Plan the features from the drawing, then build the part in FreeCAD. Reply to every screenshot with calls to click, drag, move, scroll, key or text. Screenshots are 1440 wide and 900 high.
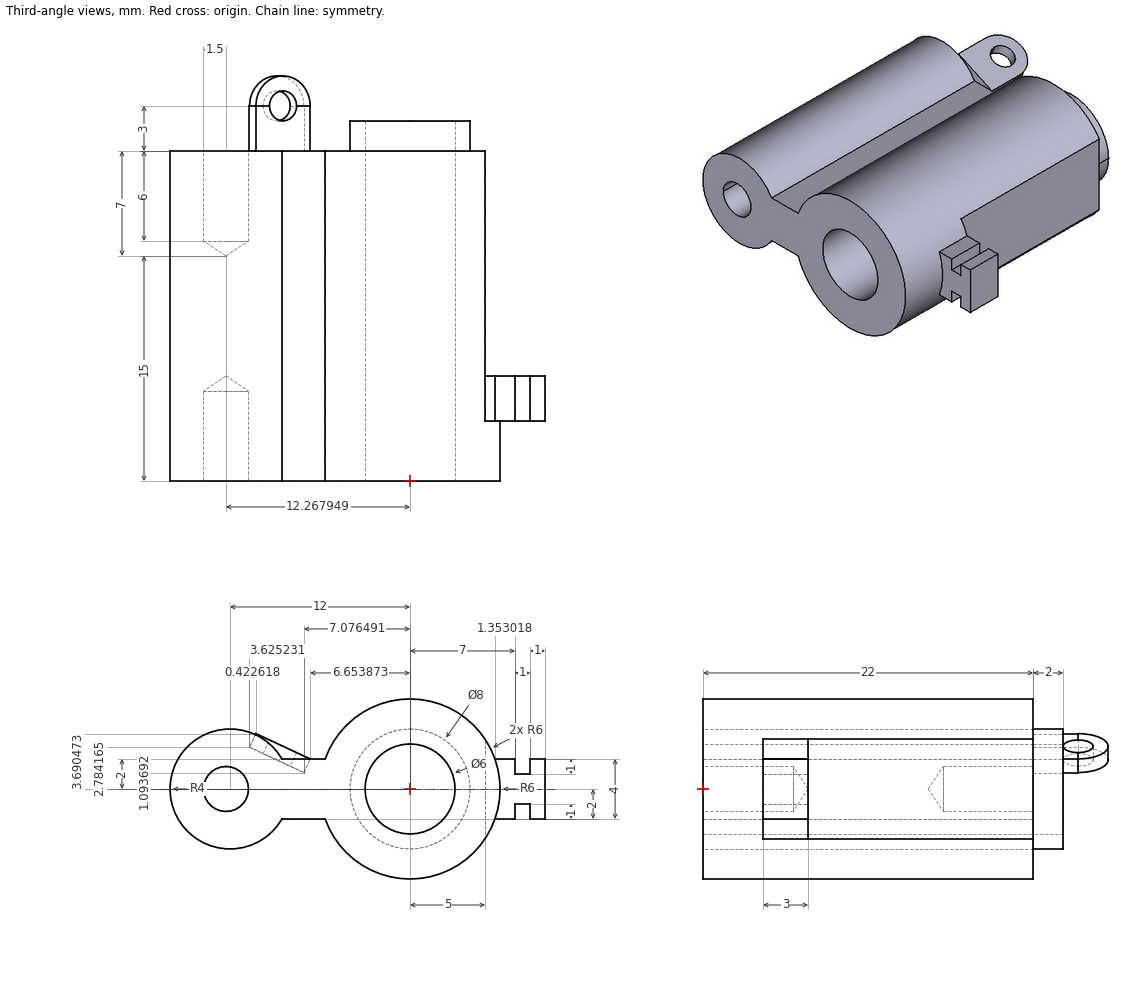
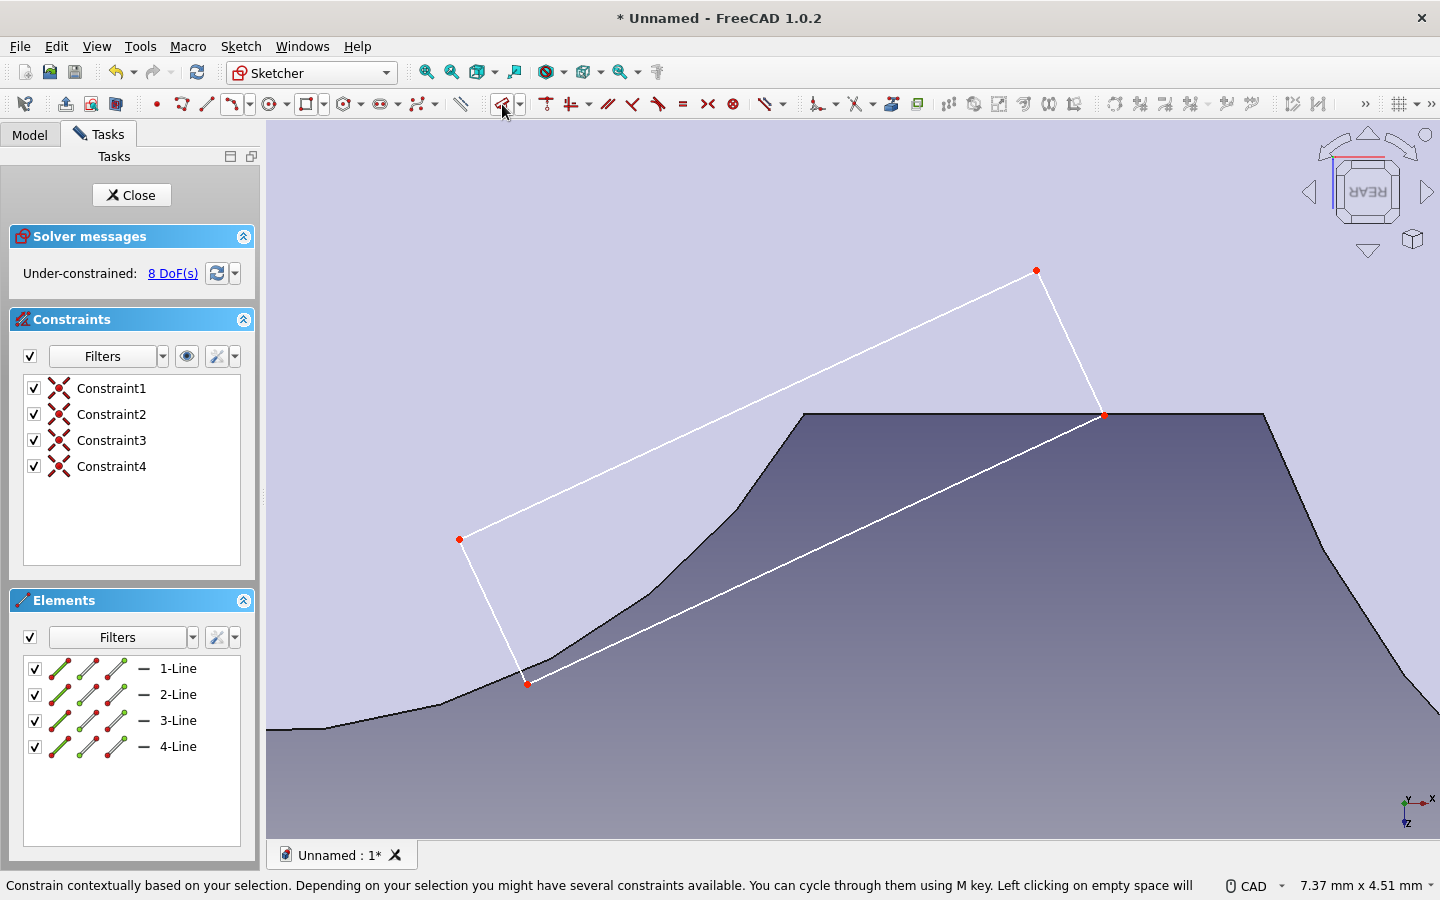
click(1104, 415)
click(1070, 282)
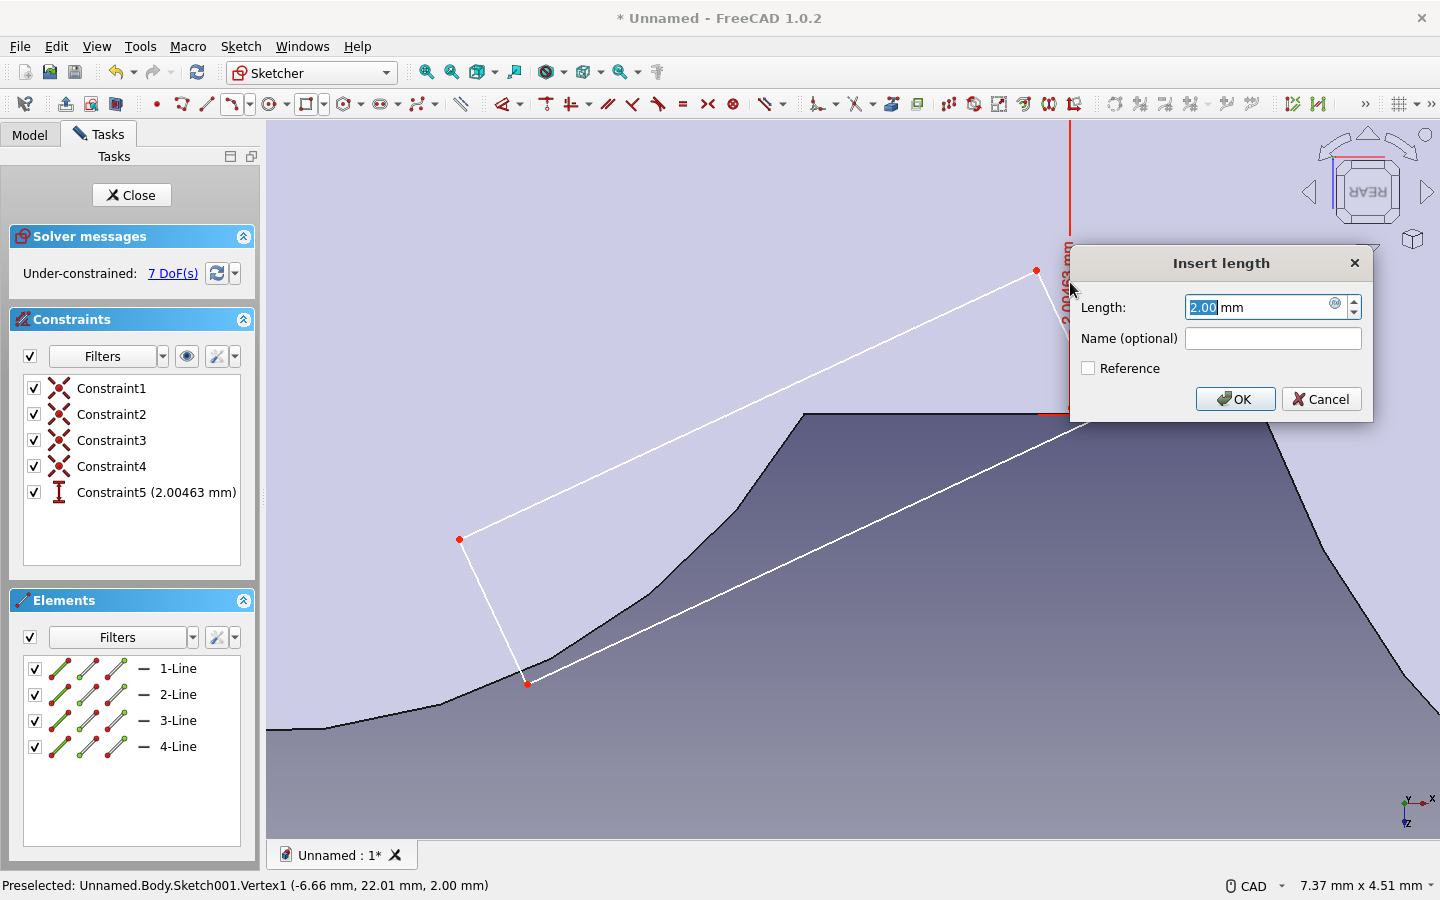
text(2)
key(Return)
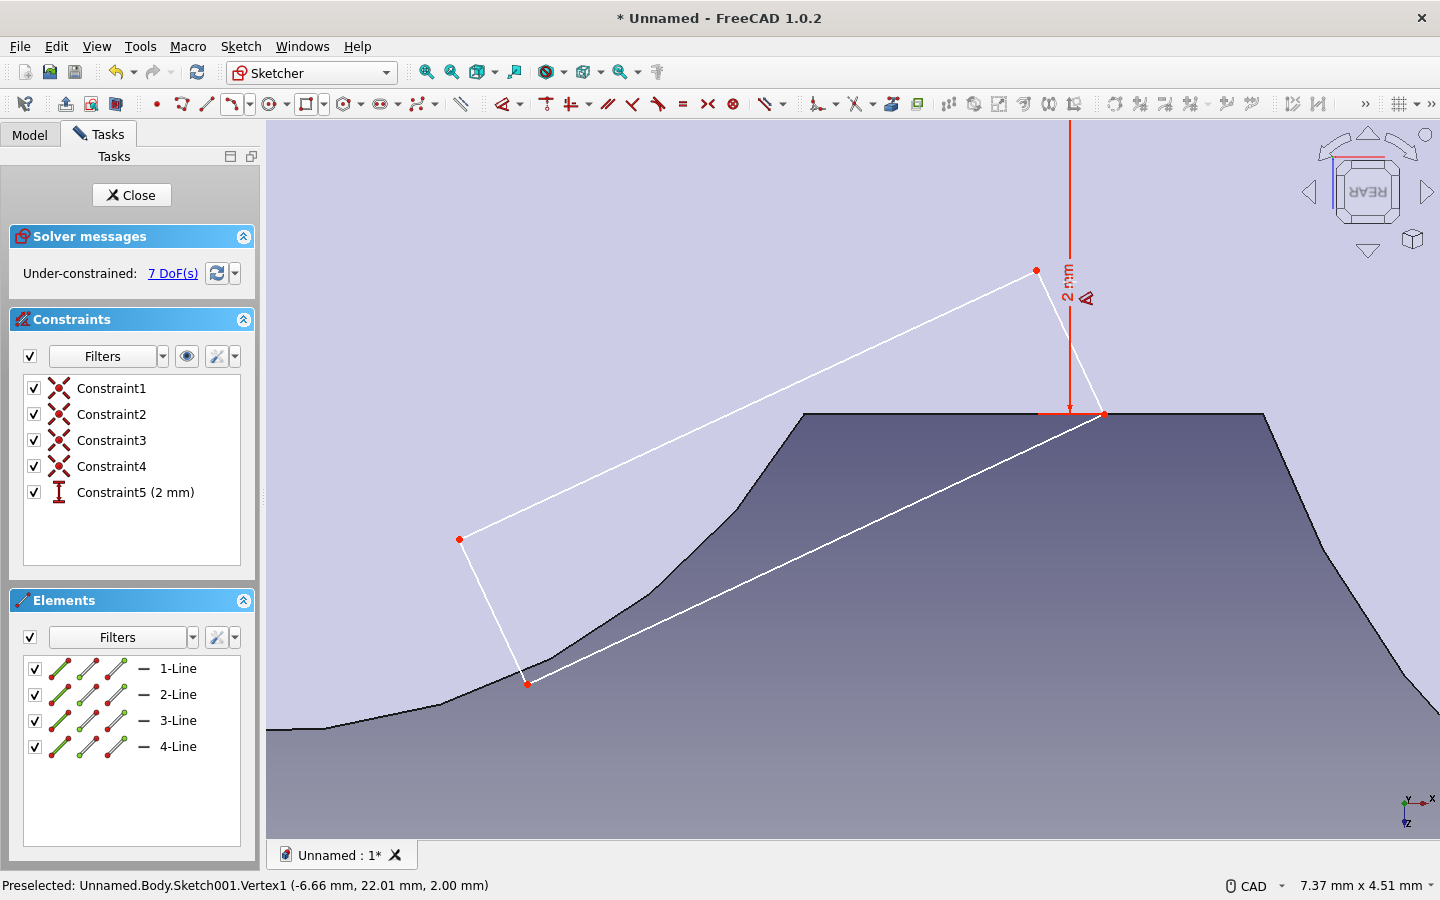
click(1104, 414)
click(1189, 448)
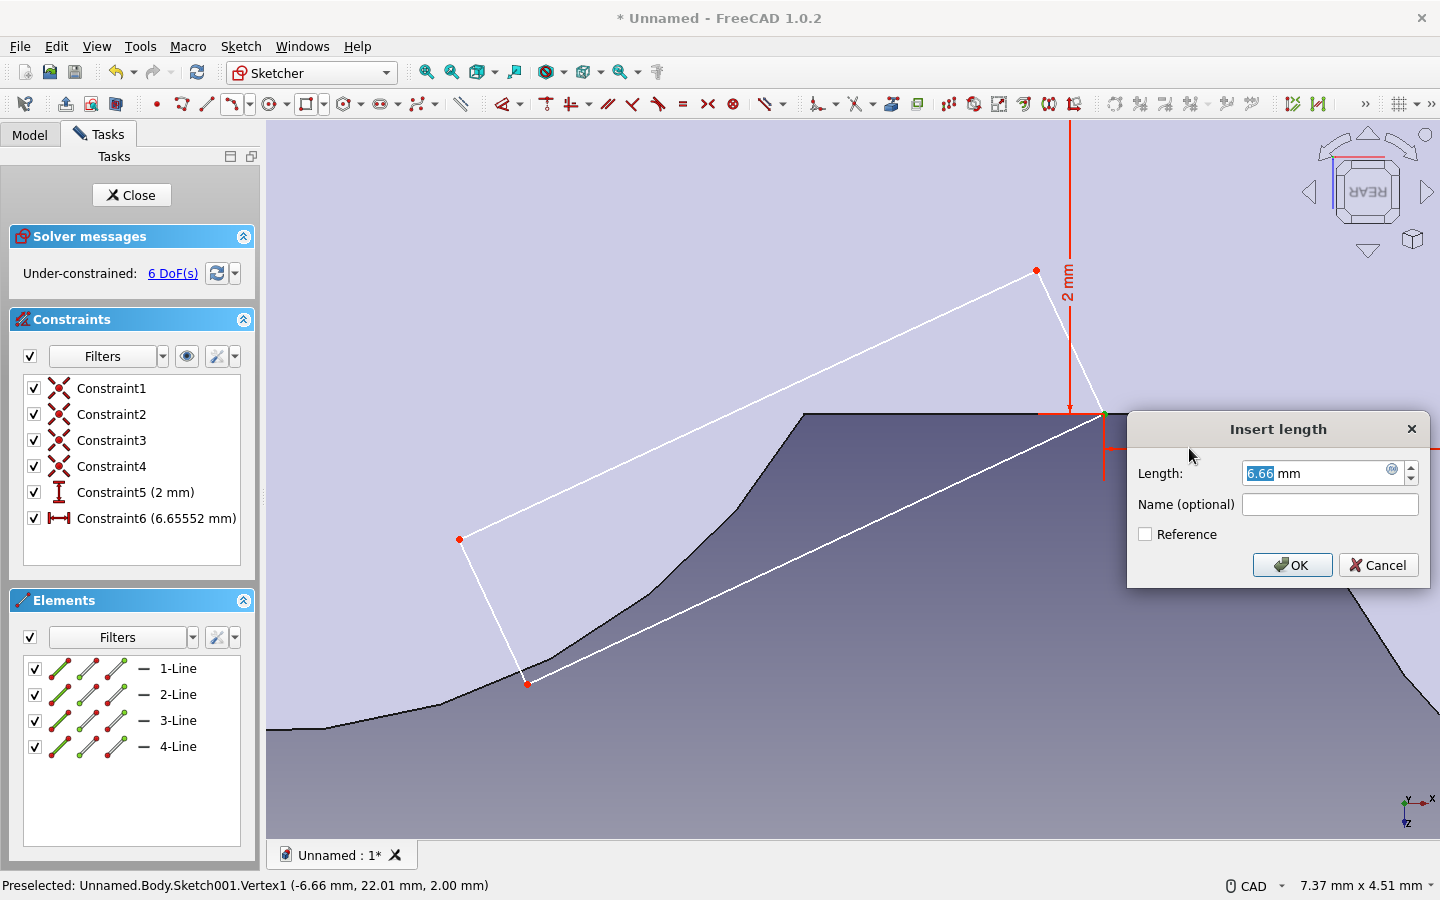
text(6.653873)
key(Return)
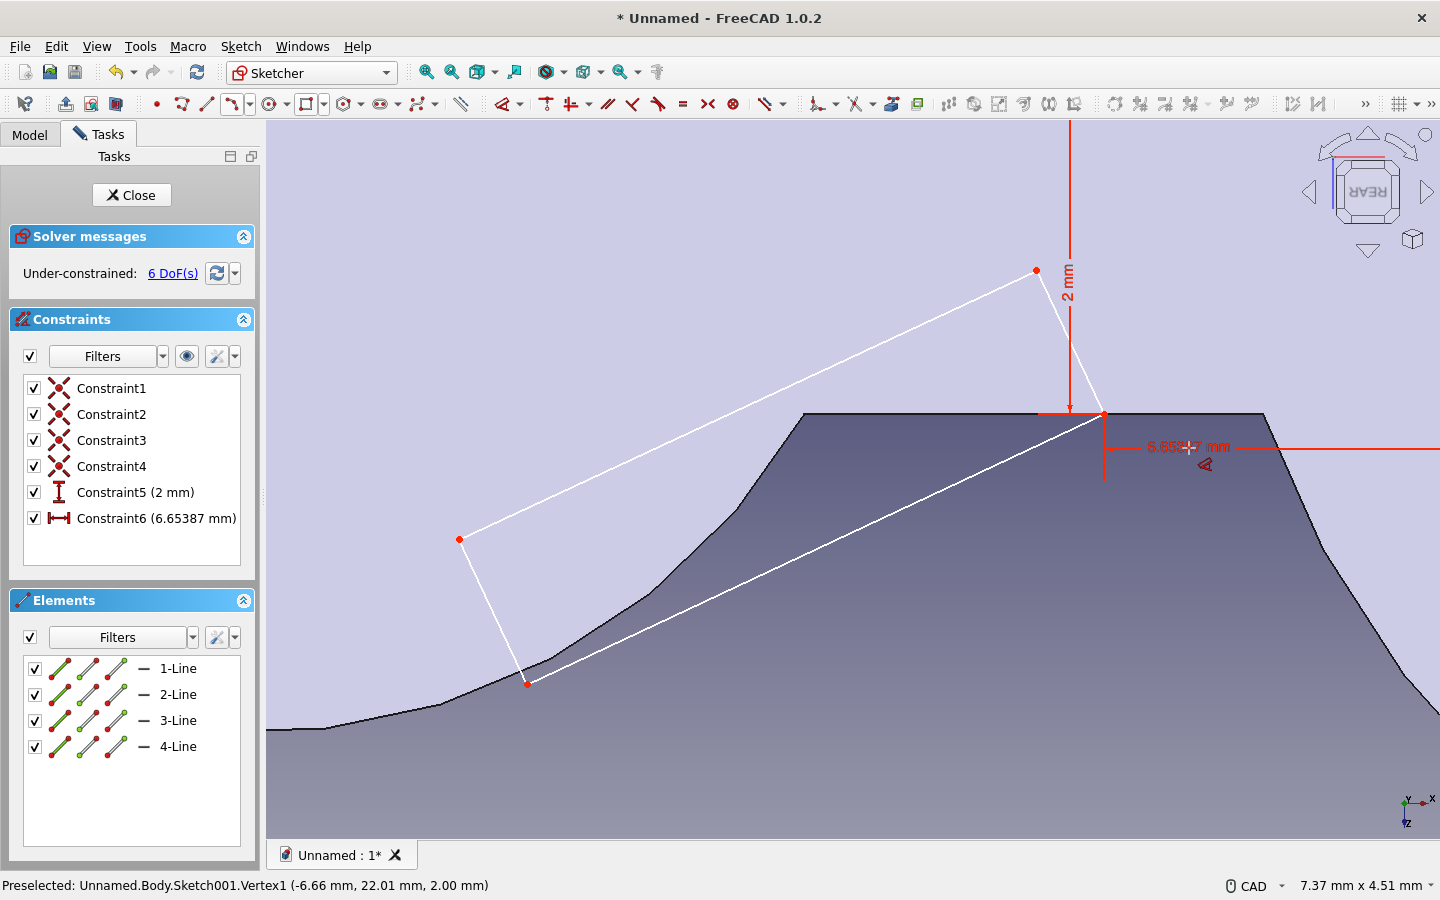
click(1037, 271)
click(1156, 305)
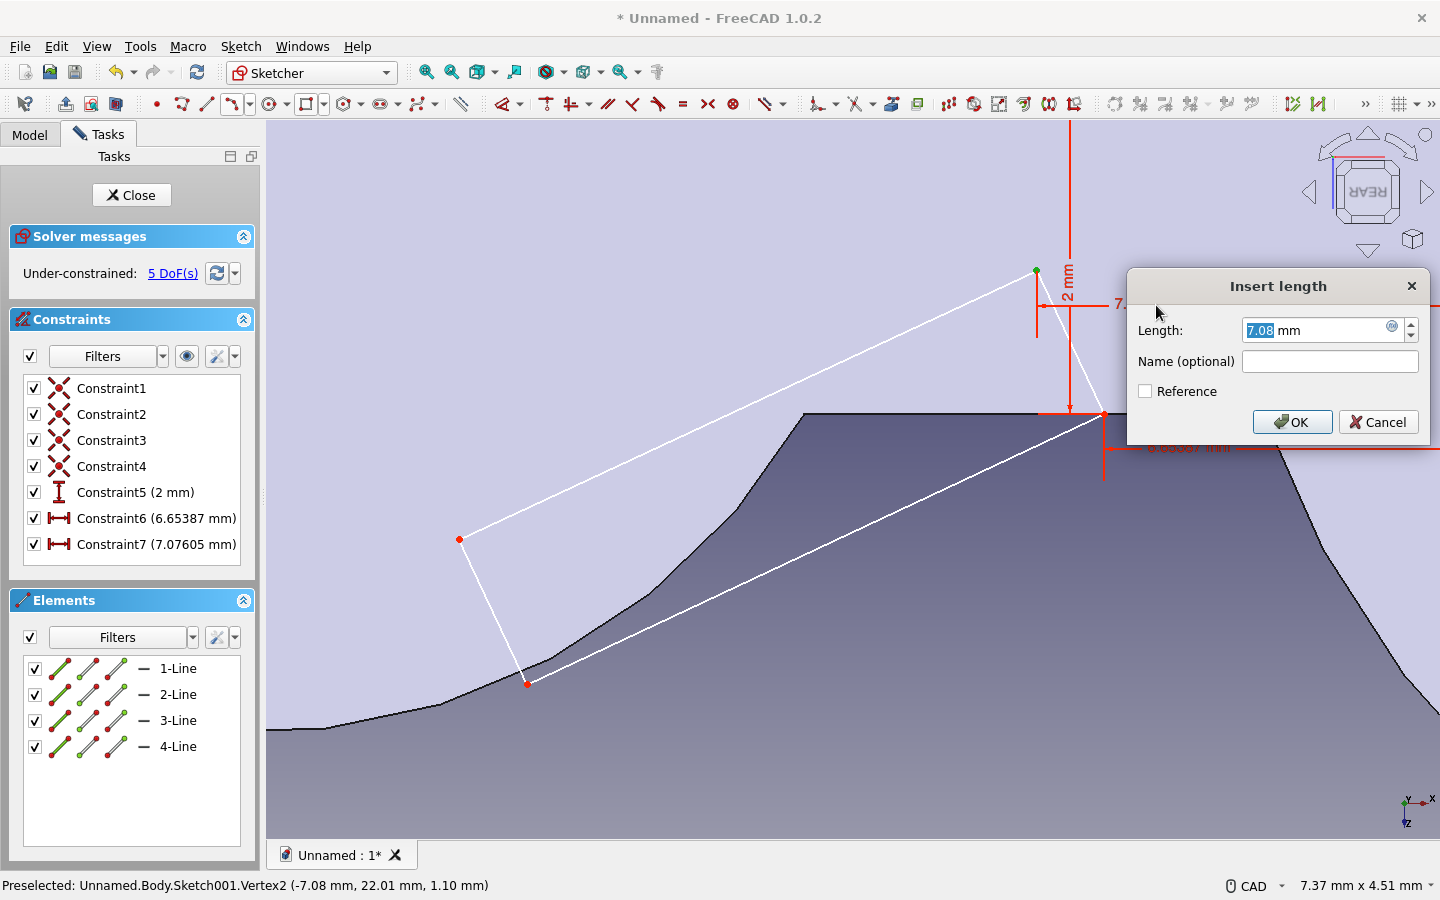
text(7.076491)
key(Return)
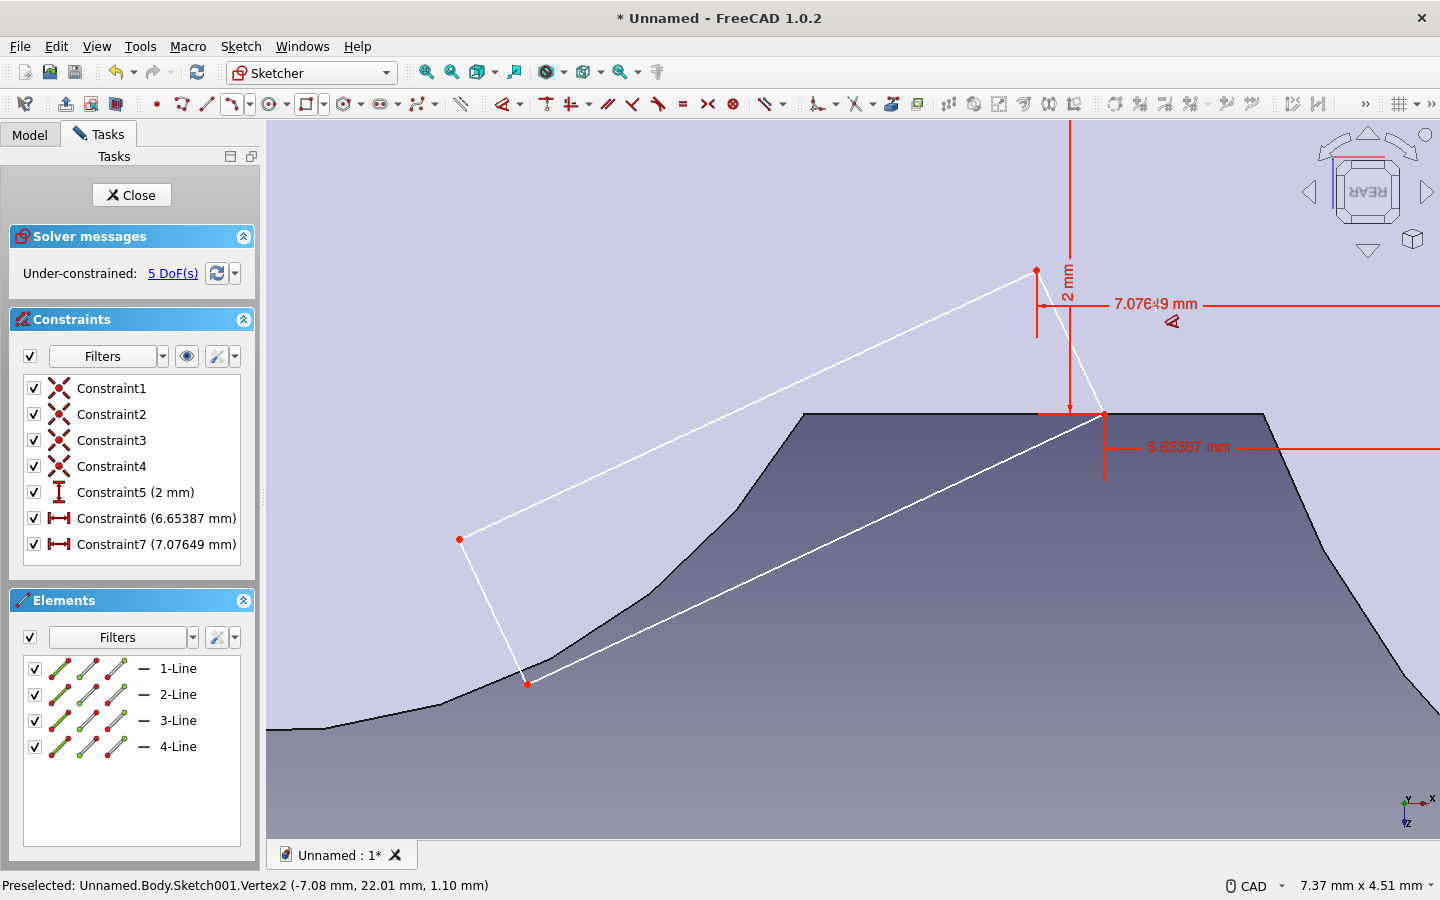
click(1037, 271)
click(1003, 210)